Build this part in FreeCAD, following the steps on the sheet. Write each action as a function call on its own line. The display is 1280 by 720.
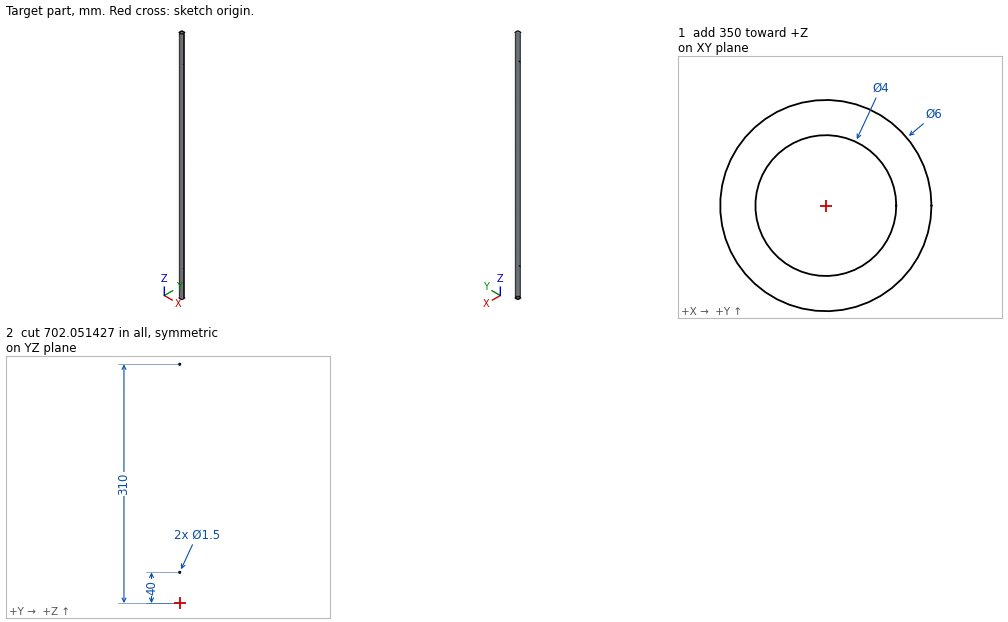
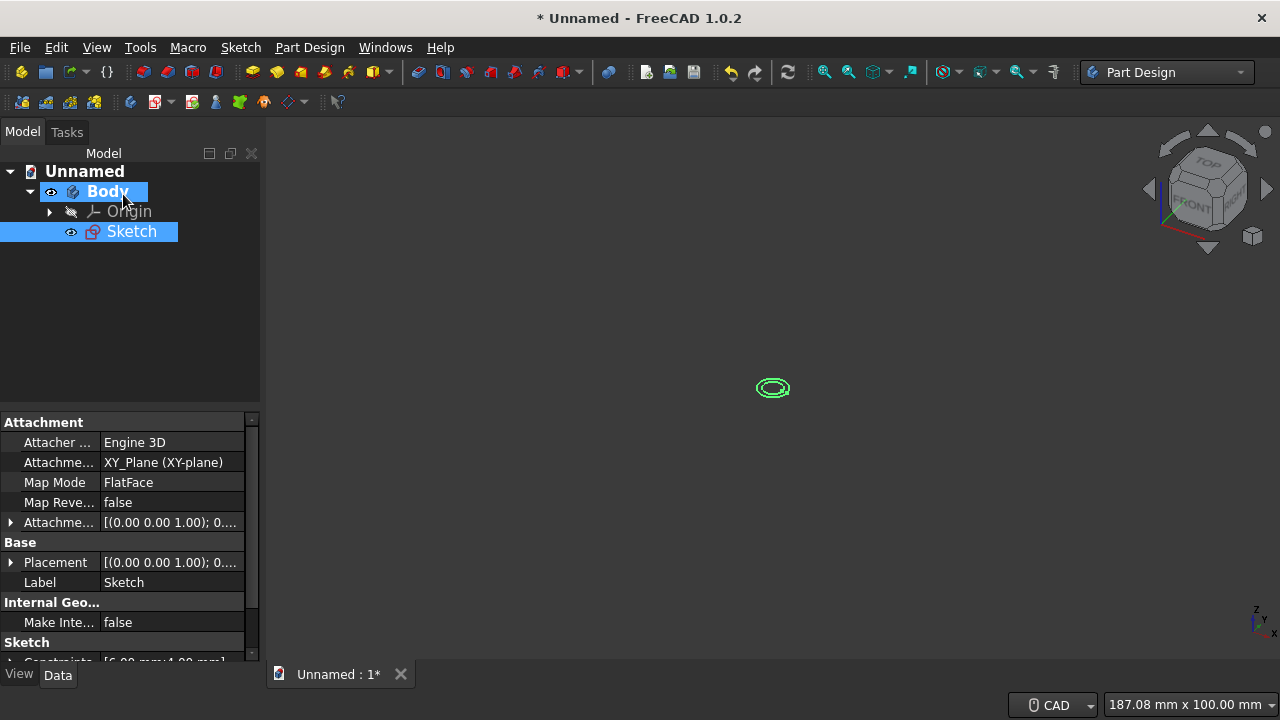
click(254, 72)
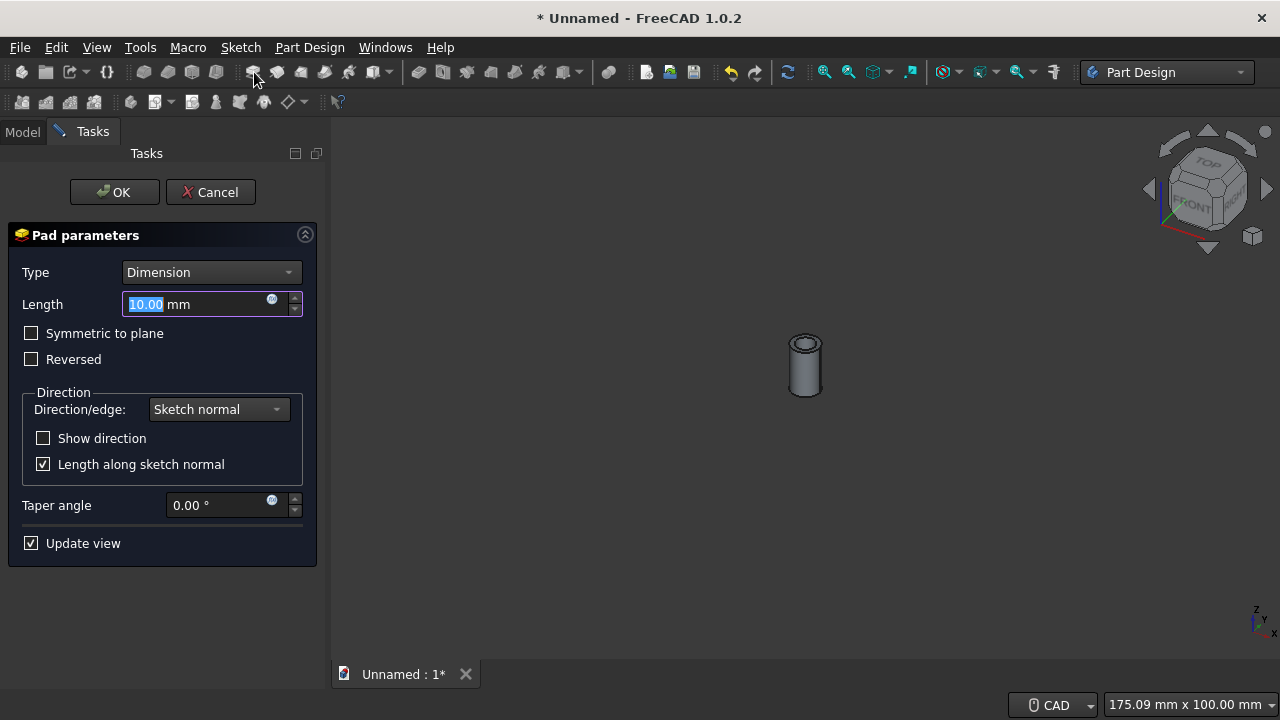
text(350)
key(Tab)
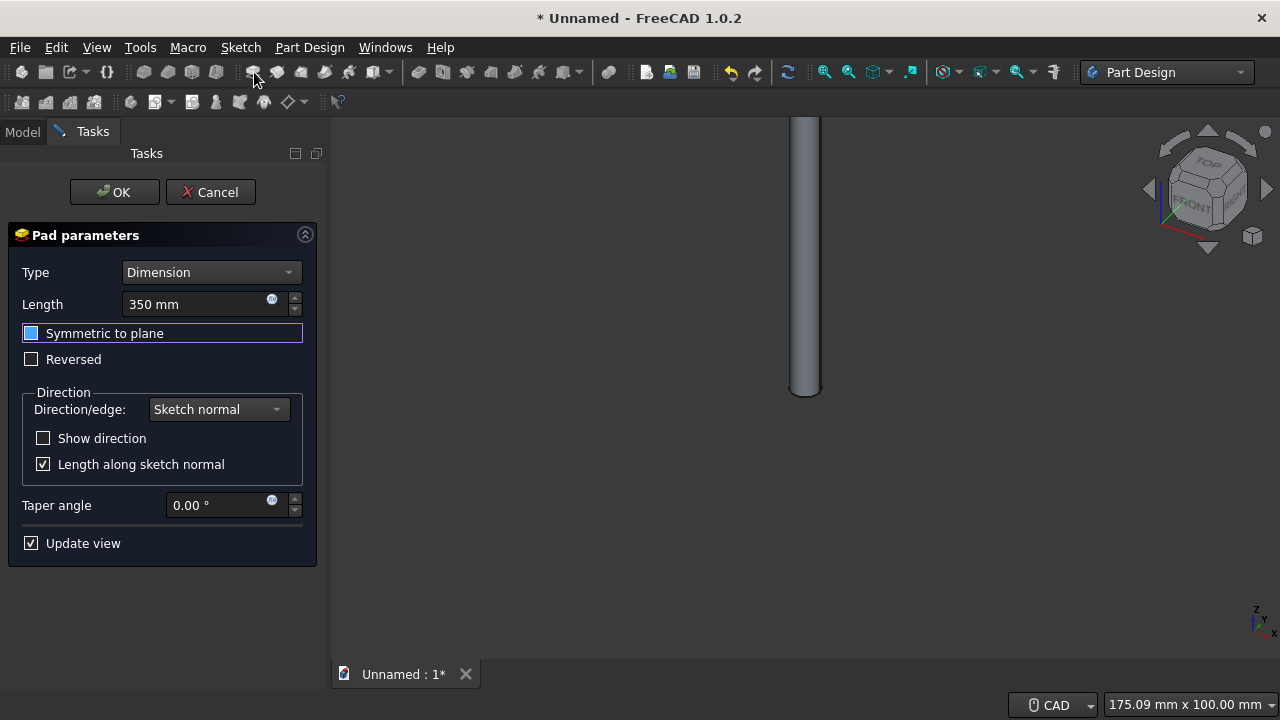
click(115, 192)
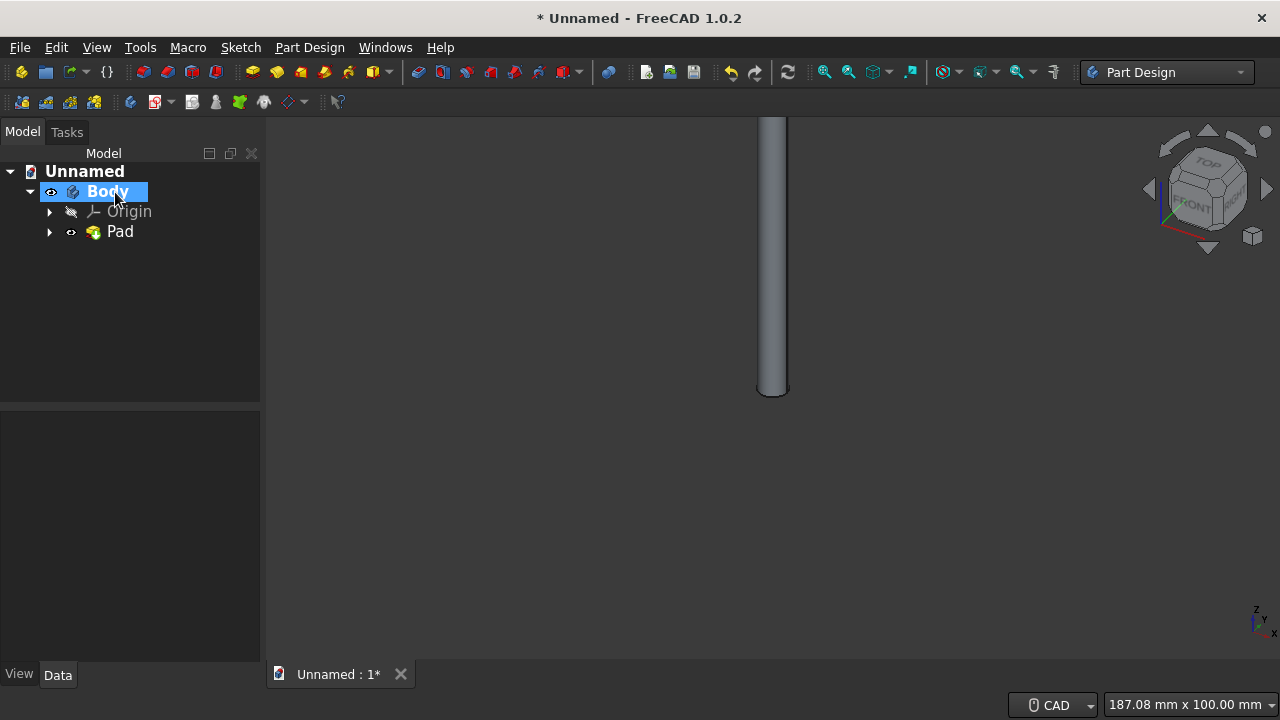
key(v)
key(f)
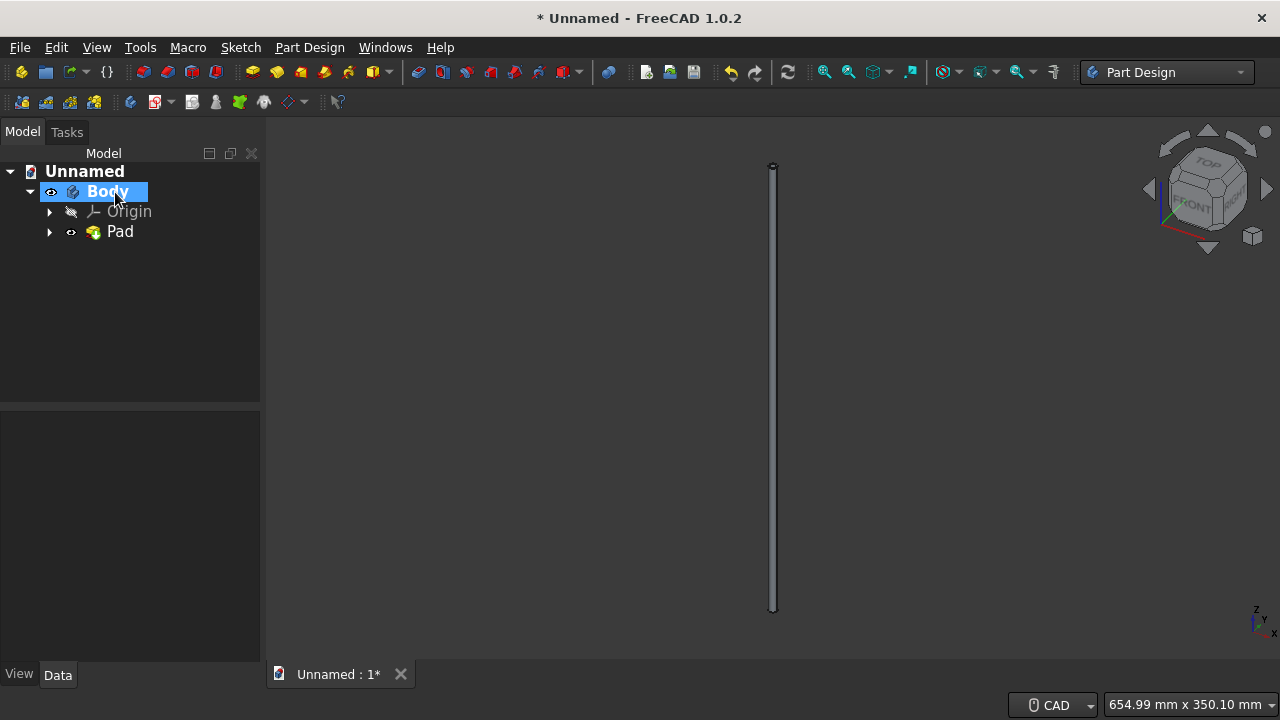
click(156, 102)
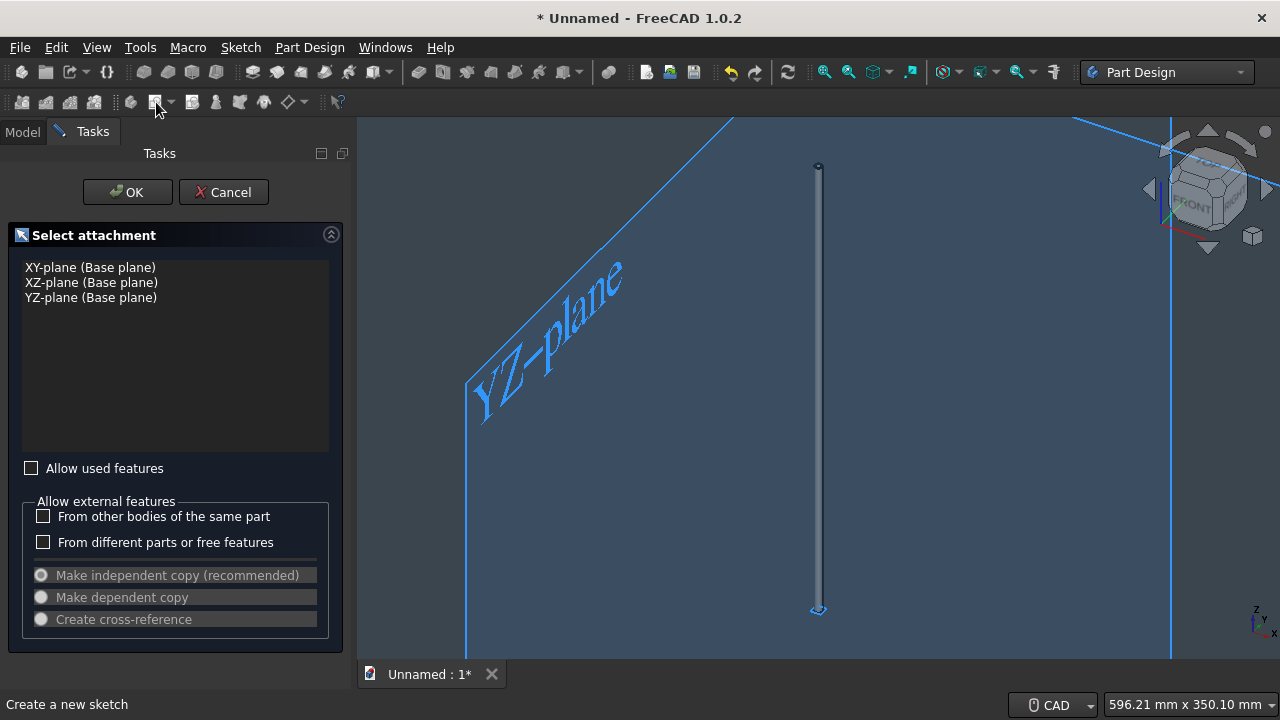
click(82, 298)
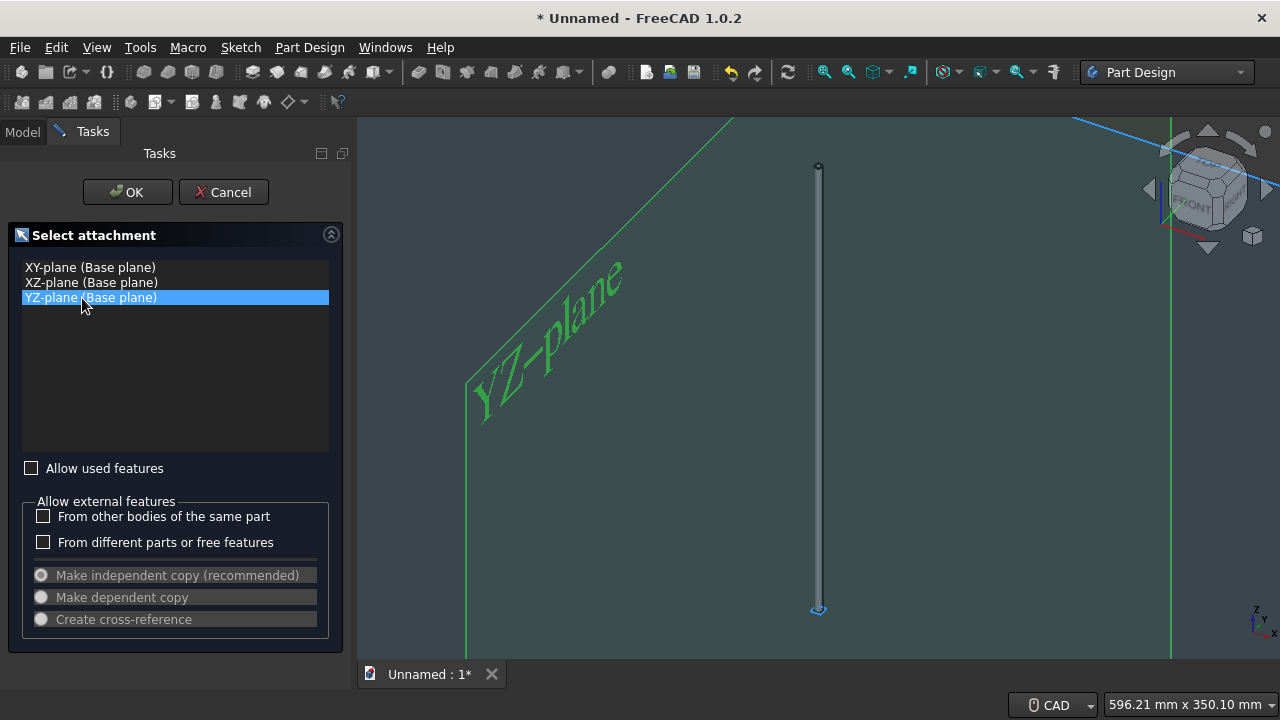
click(128, 192)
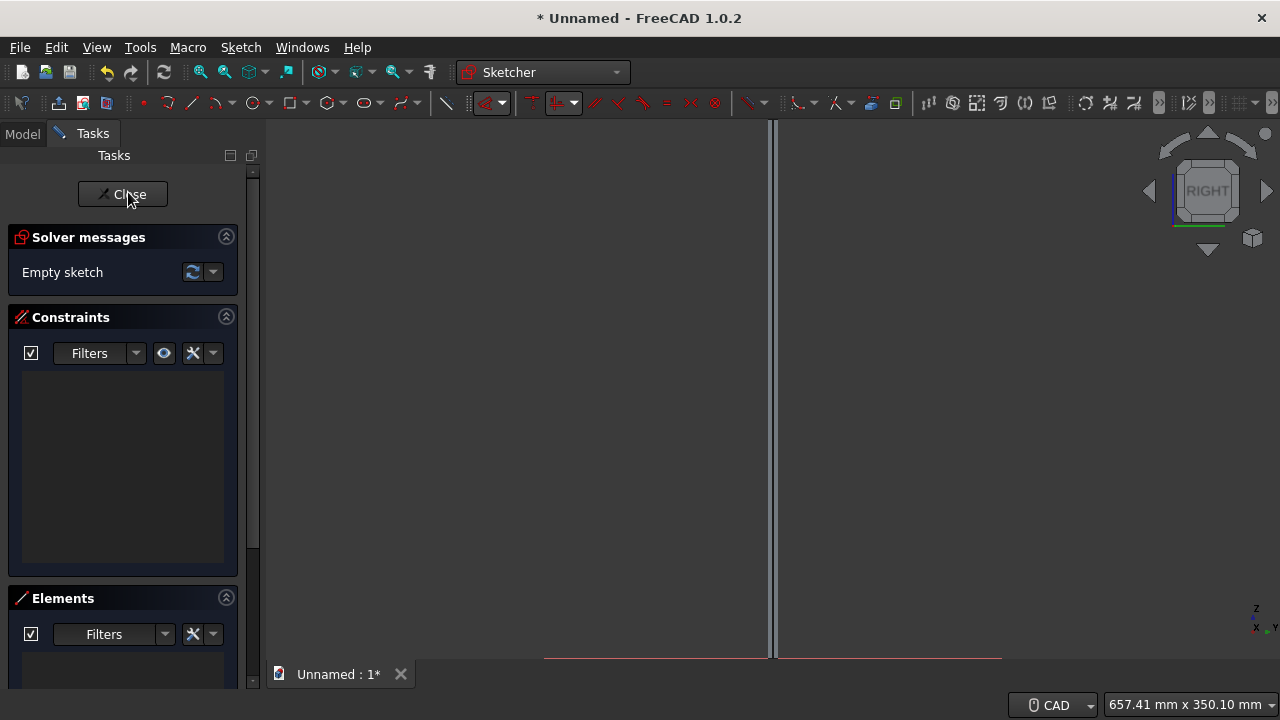
click(108, 104)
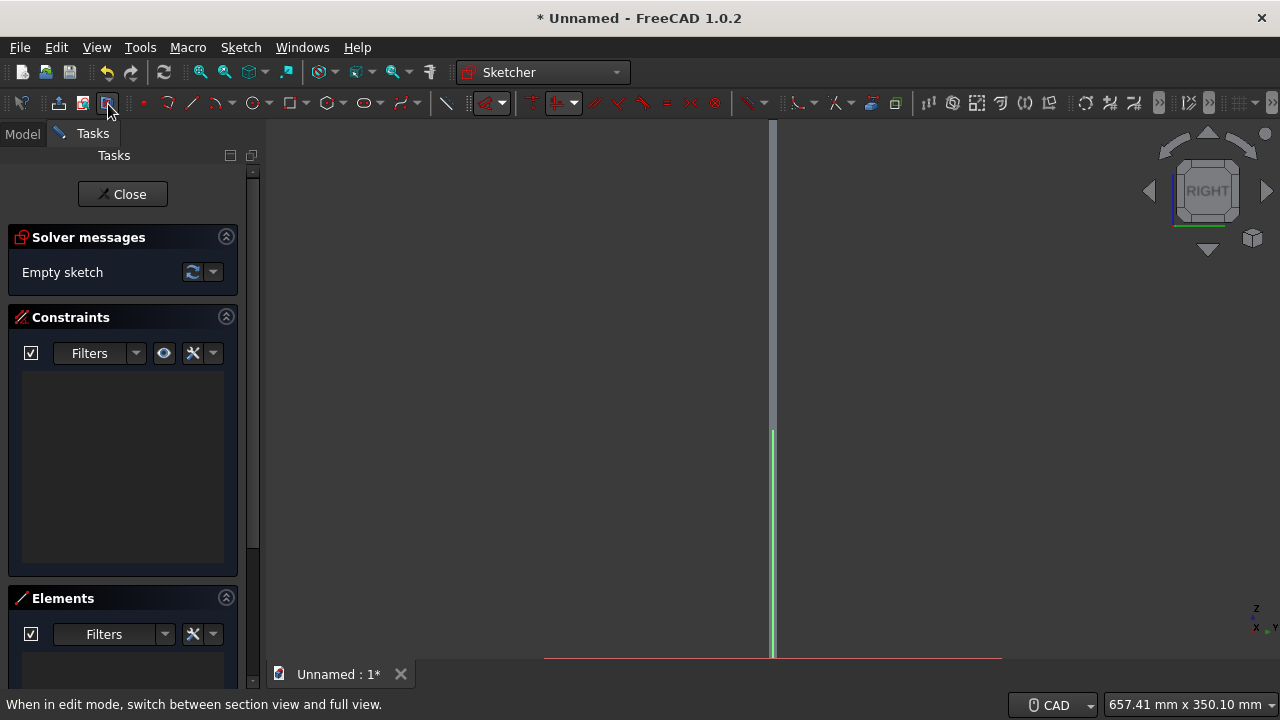
scroll(565, 327, down, 2)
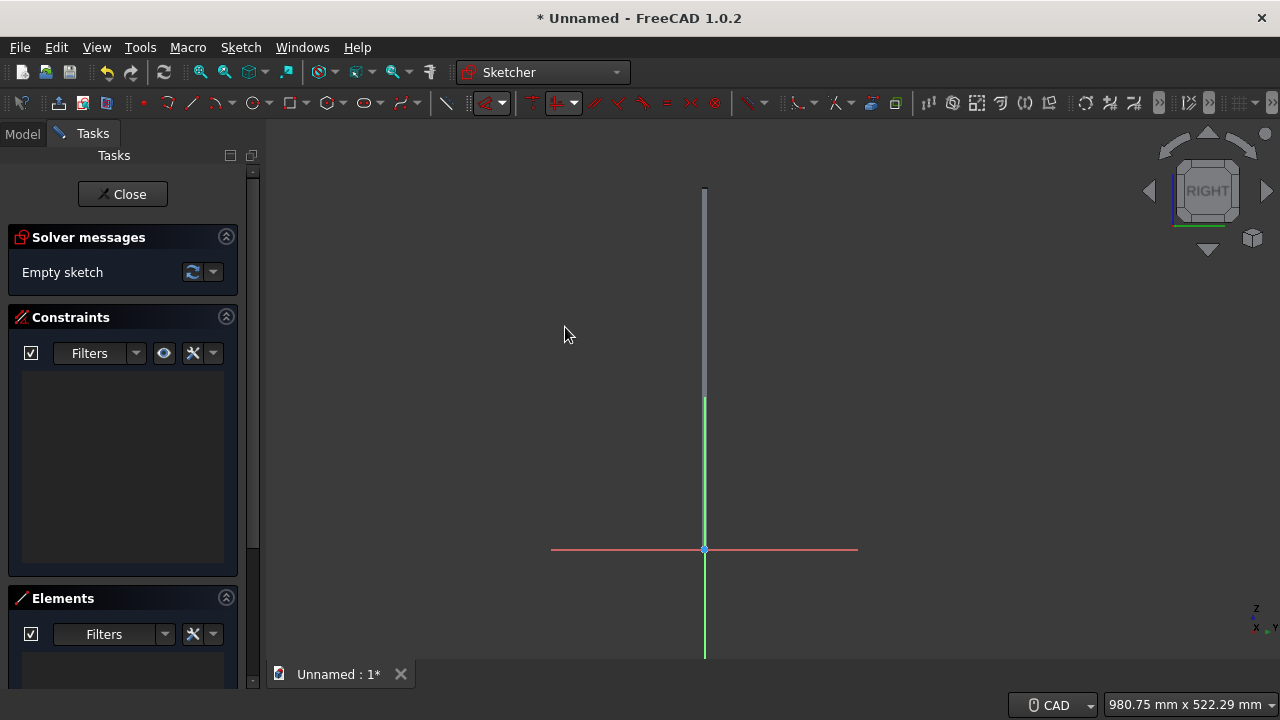
key(g)
key(c)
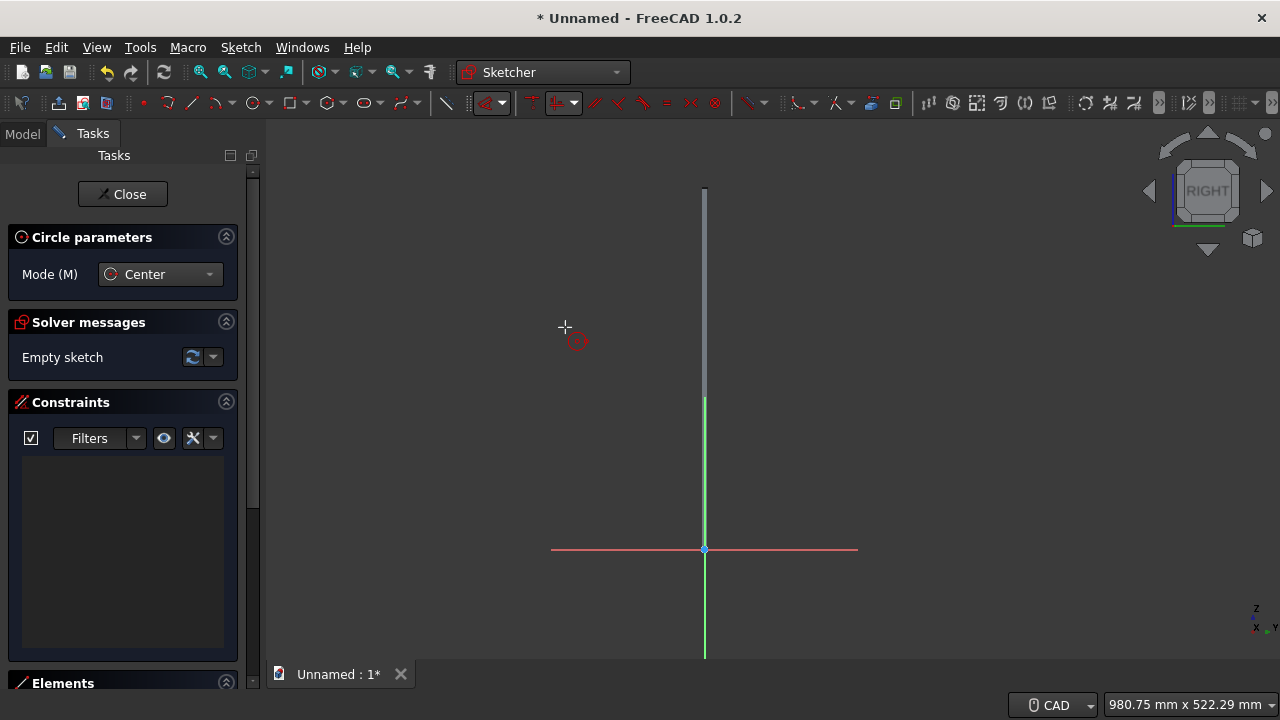
scroll(705, 508, up, 17)